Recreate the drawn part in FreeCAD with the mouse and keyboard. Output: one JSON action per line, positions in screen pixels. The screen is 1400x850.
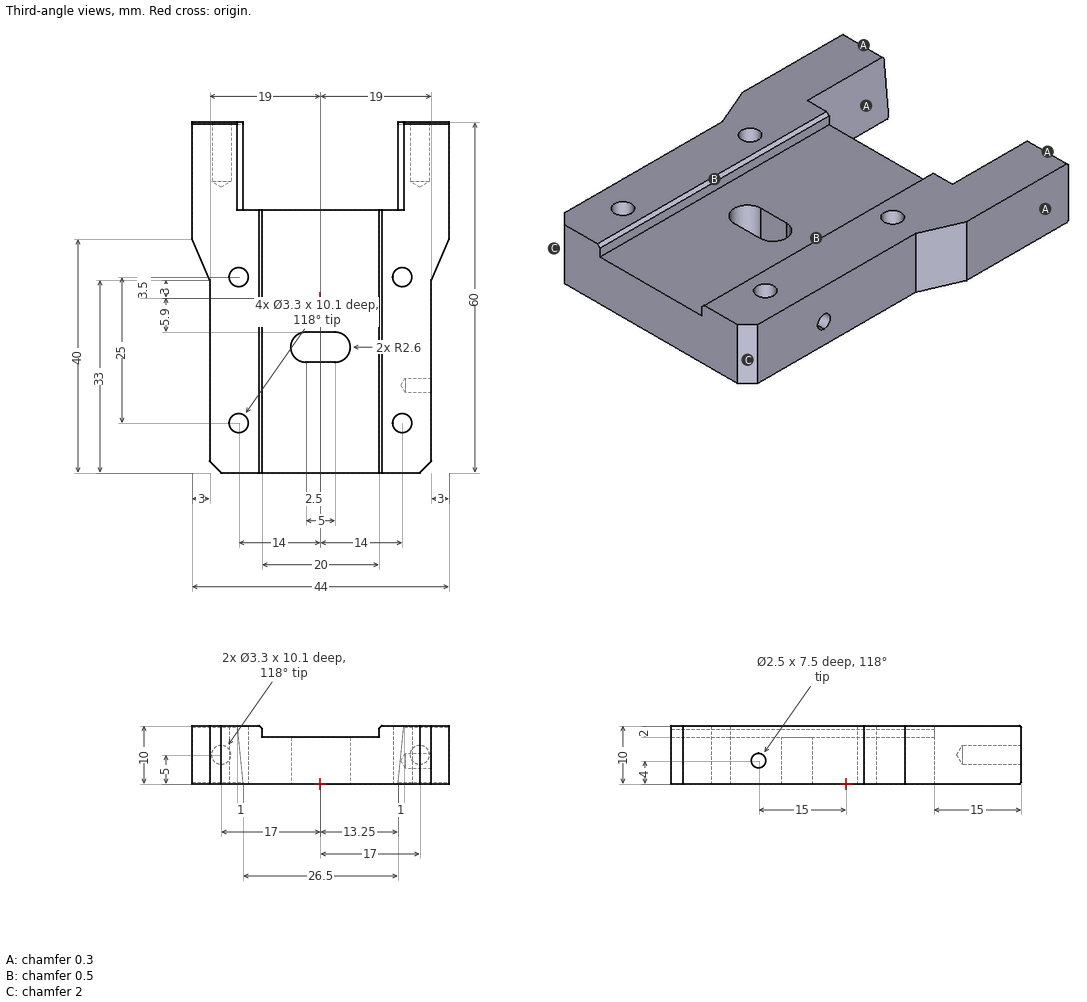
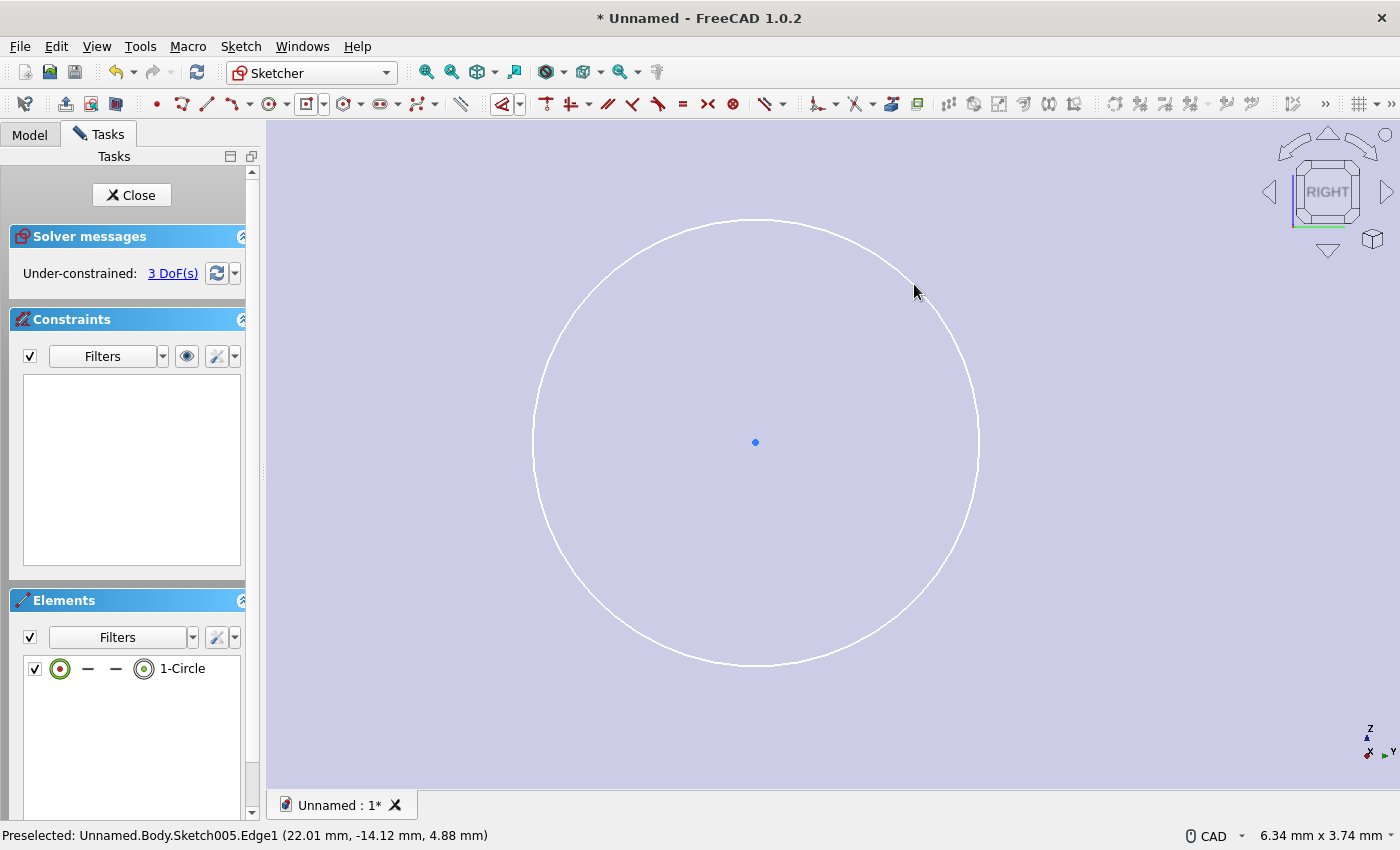
{"action": "left_click", "coordinate": [914, 285]}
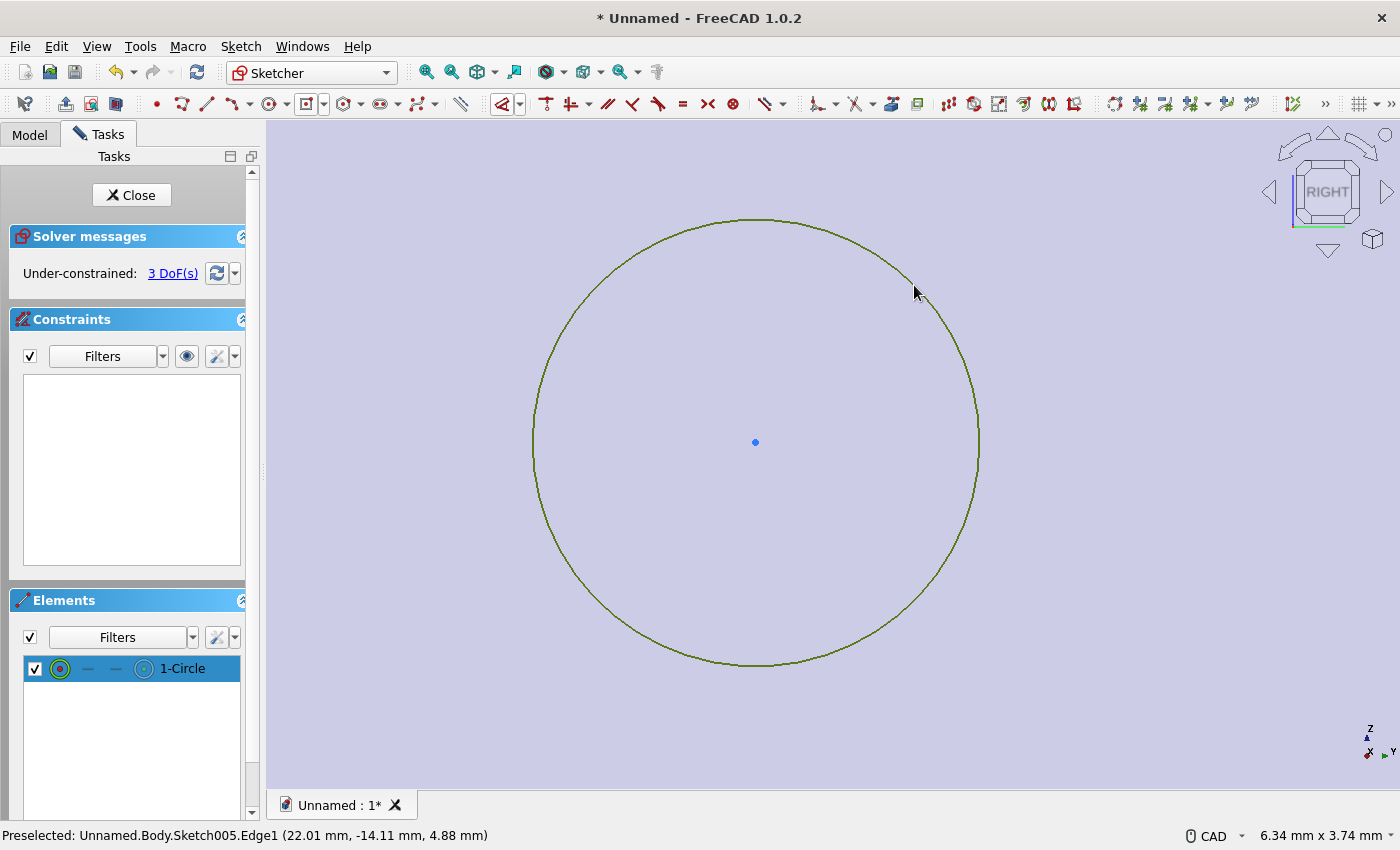
{"action": "key", "text": "k o"}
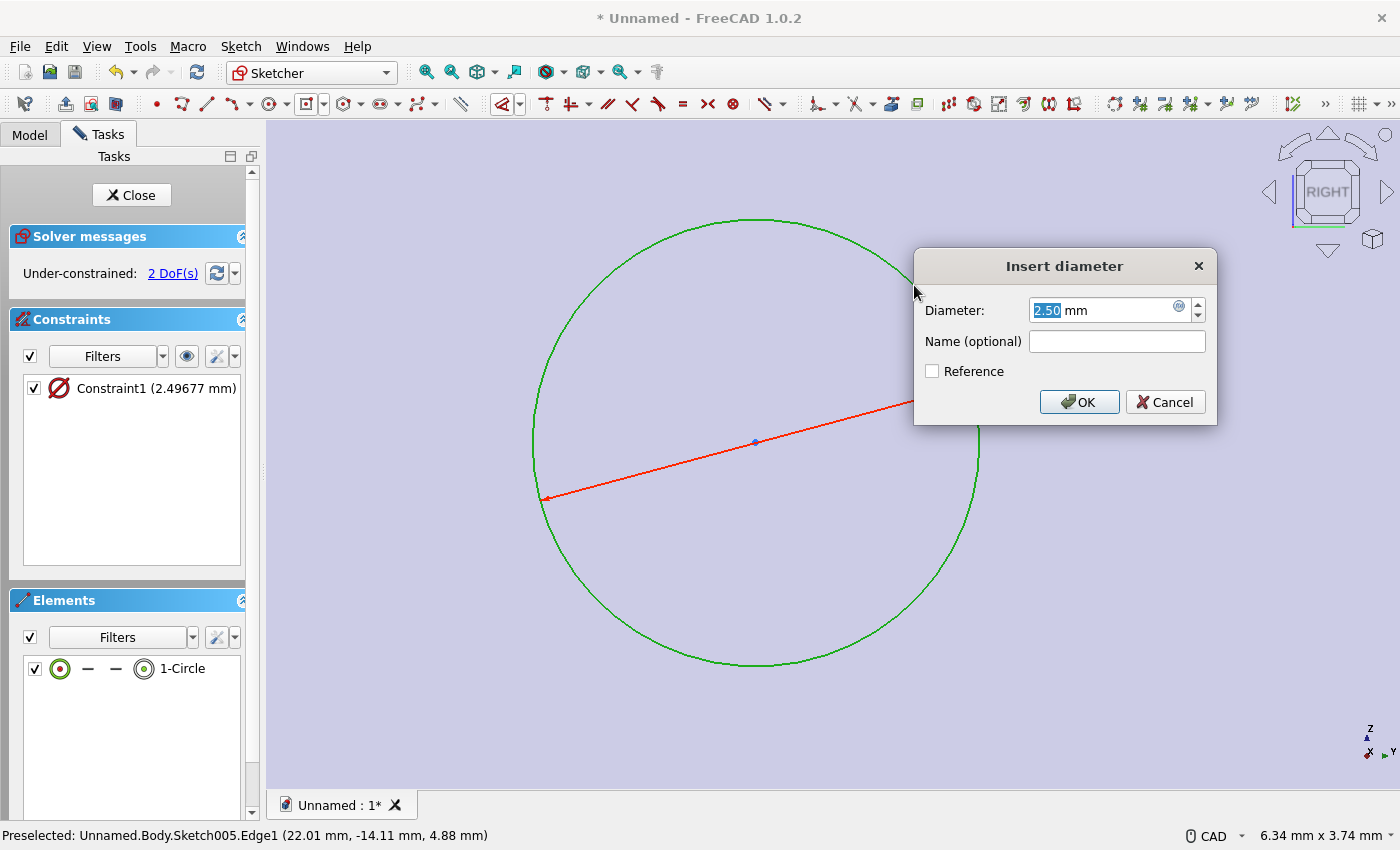
{"action": "type", "text": "2.5"}
{"action": "key", "text": "Return"}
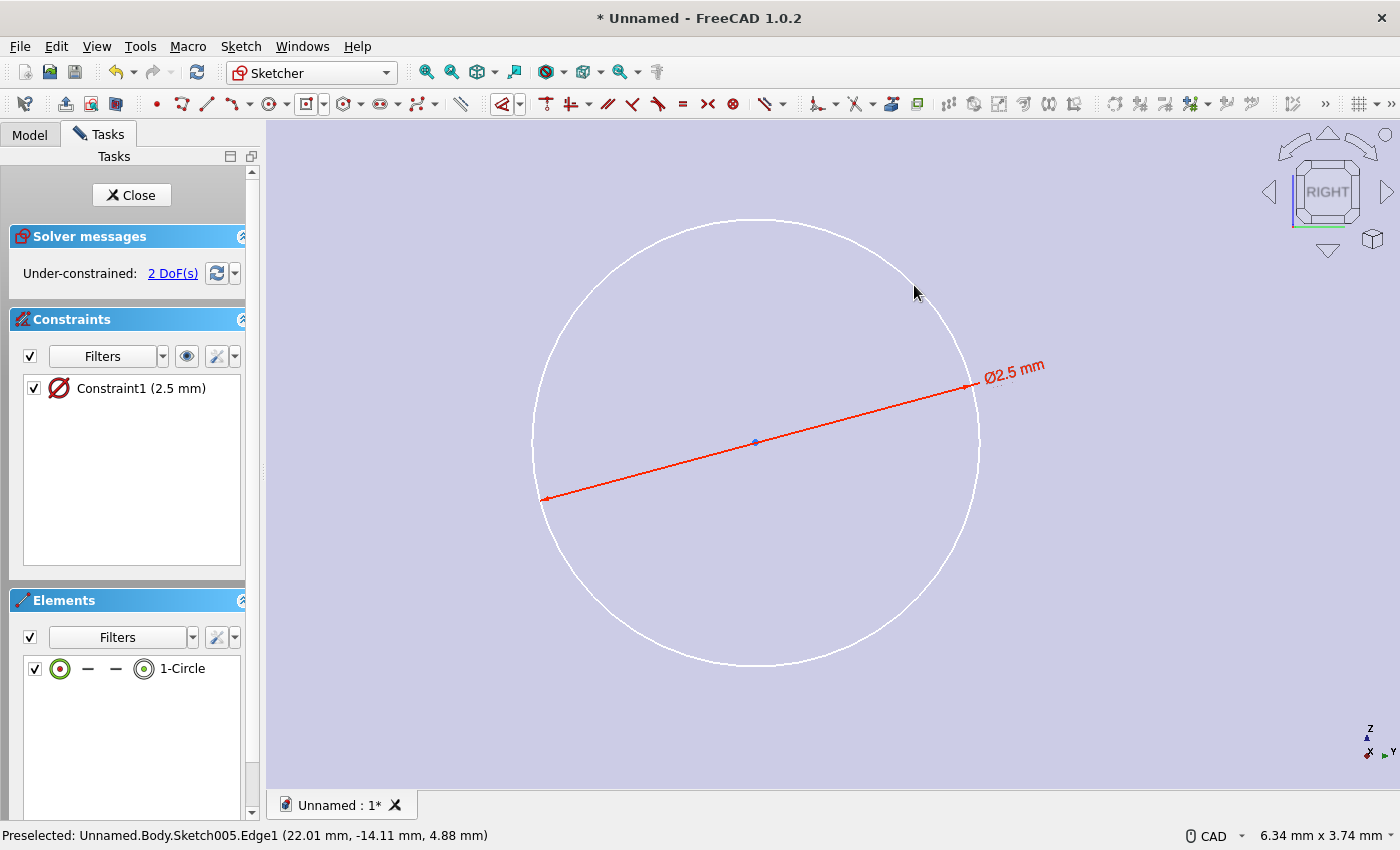
{"action": "left_click", "coordinate": [756, 443]}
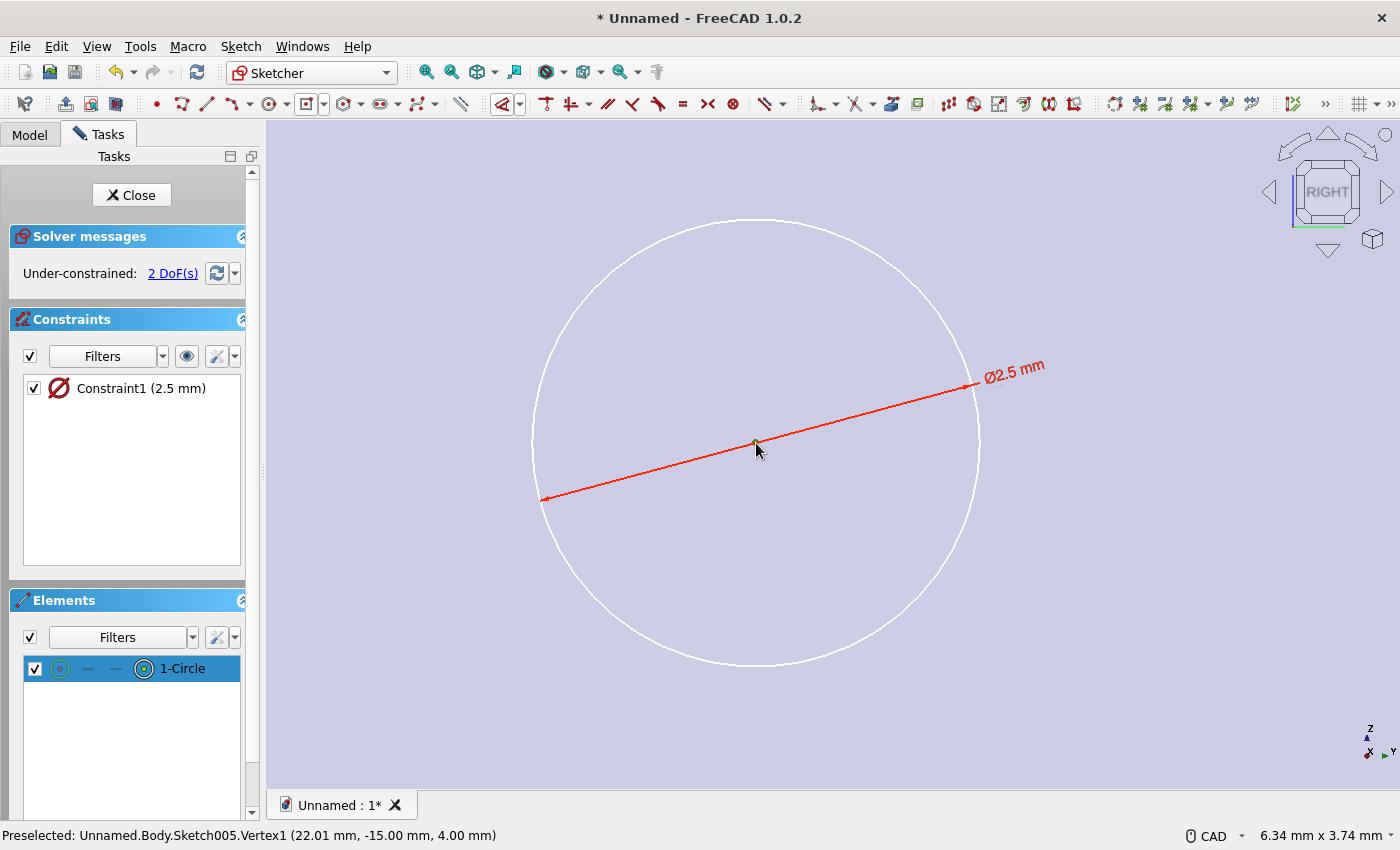
{"action": "left_click", "coordinate": [520, 104]}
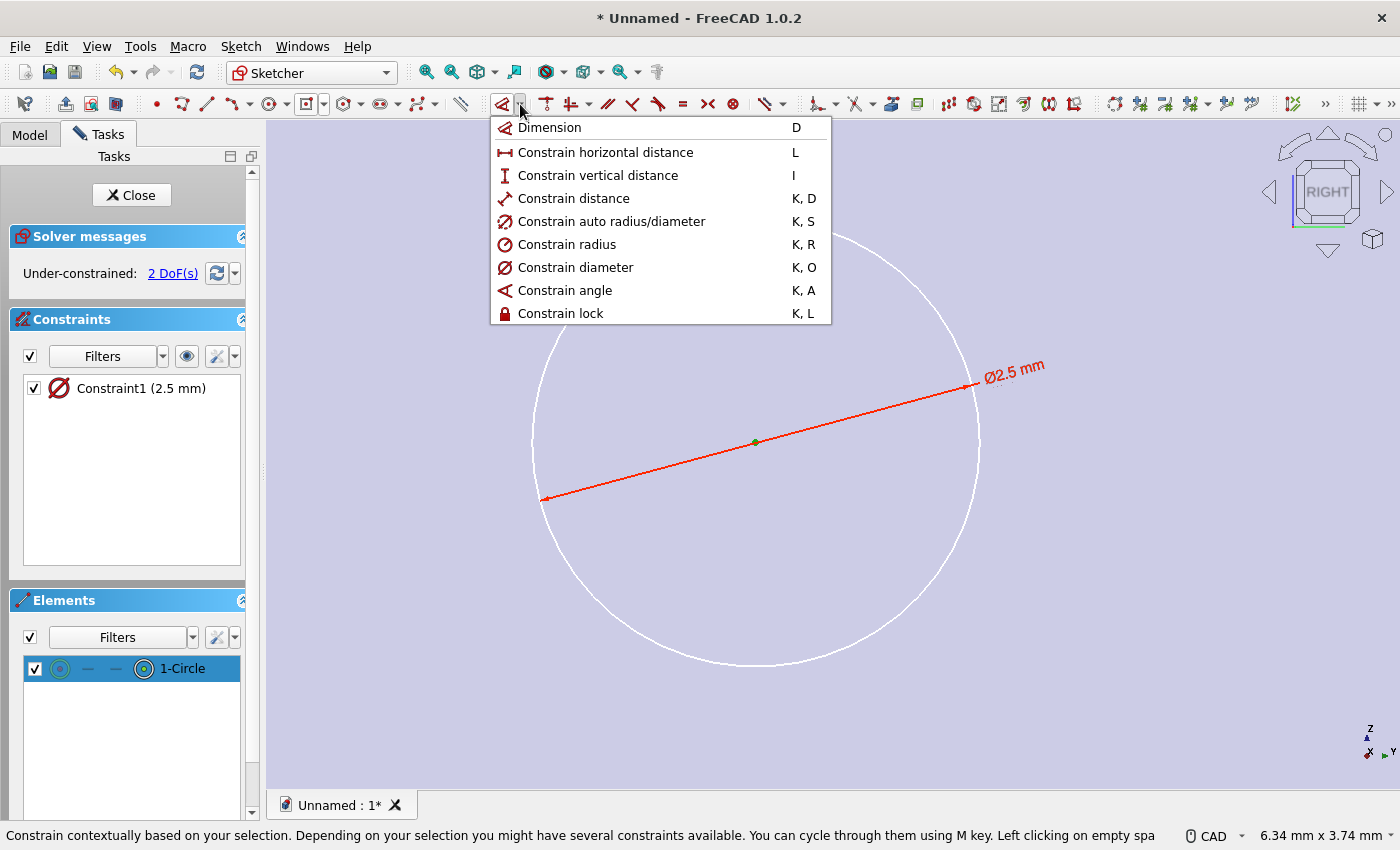
{"action": "left_click", "coordinate": [661, 176]}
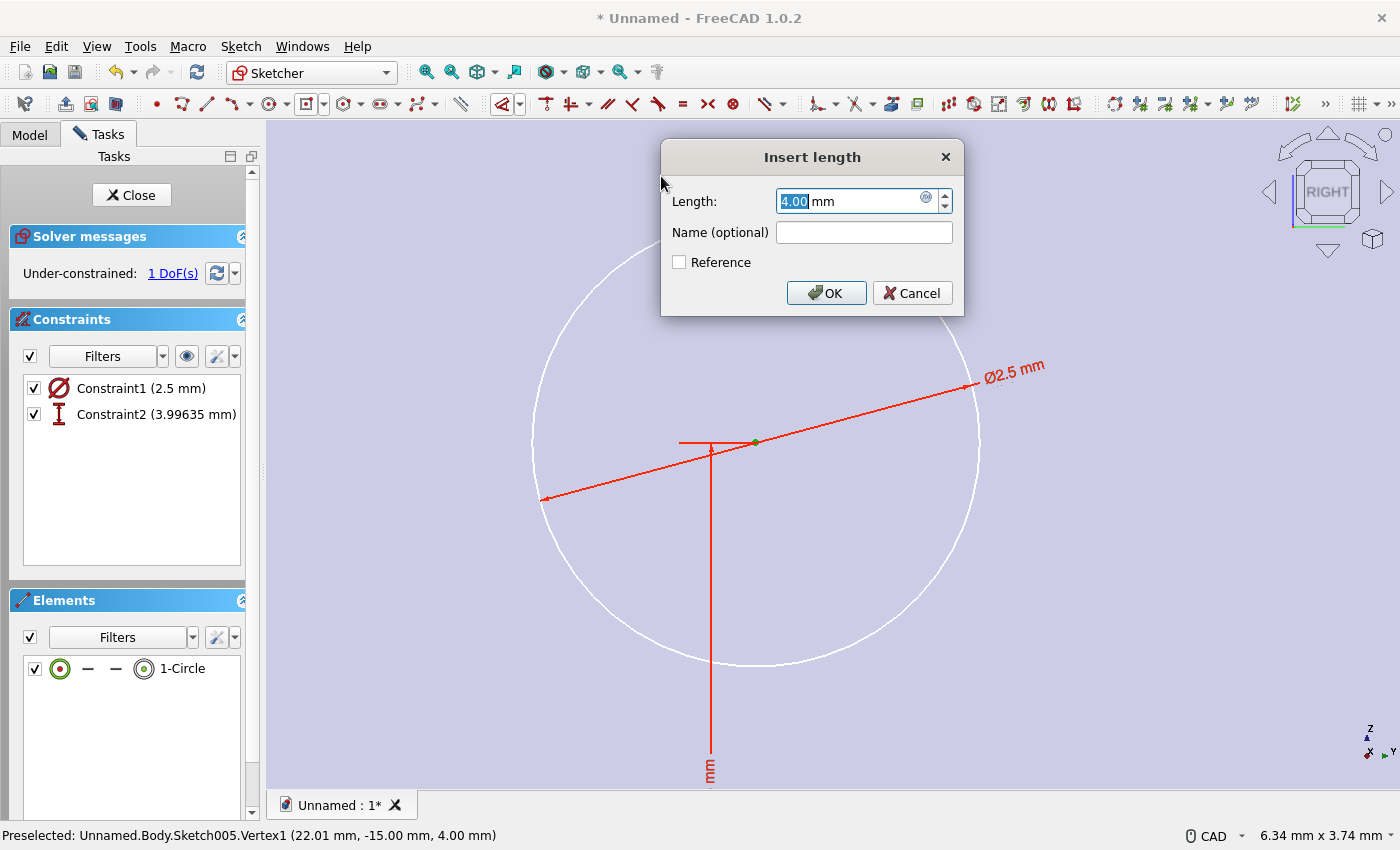
{"action": "type", "text": "4"}
{"action": "key", "text": "Return"}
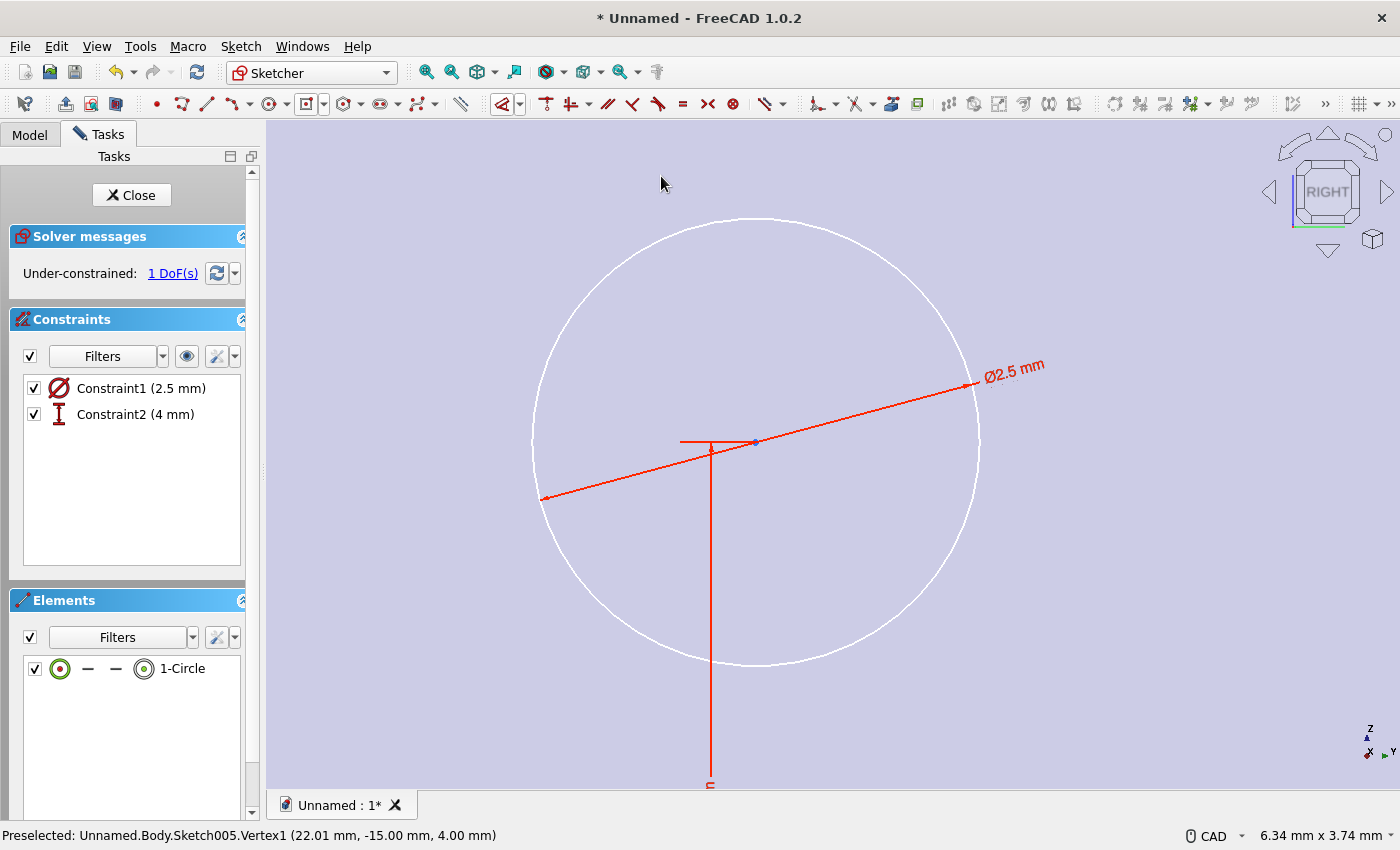
{"action": "left_click", "coordinate": [756, 442]}